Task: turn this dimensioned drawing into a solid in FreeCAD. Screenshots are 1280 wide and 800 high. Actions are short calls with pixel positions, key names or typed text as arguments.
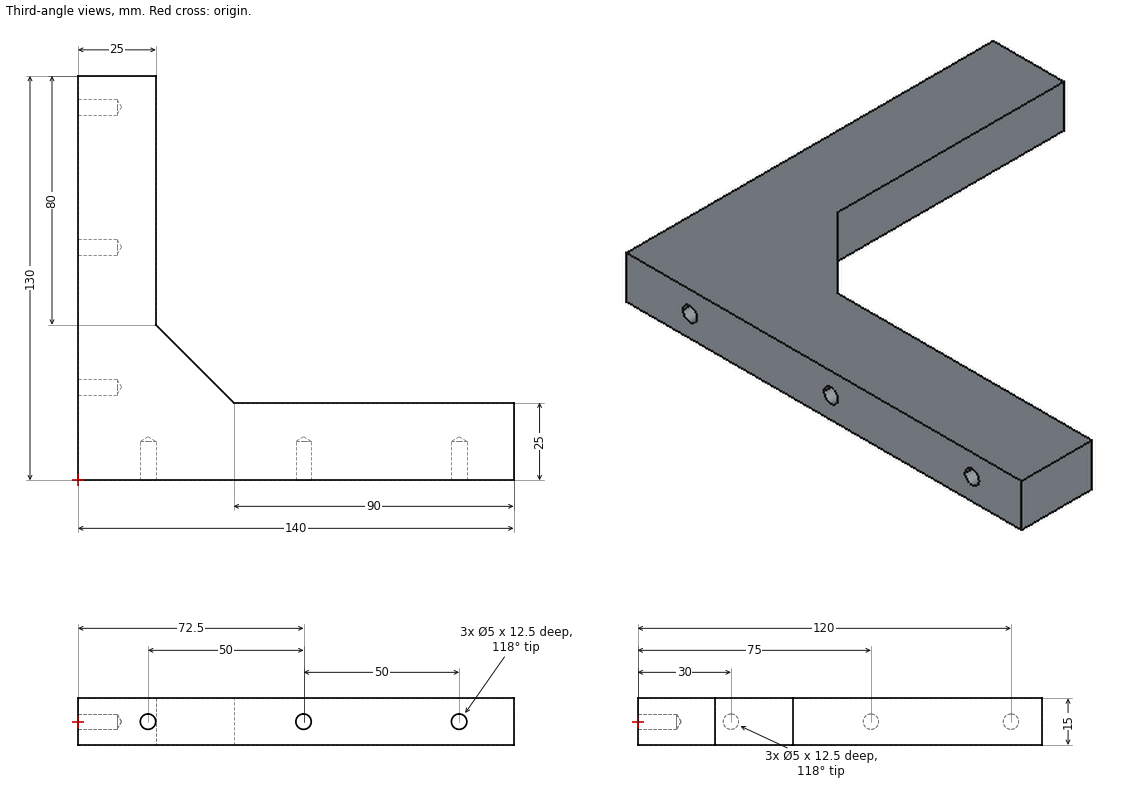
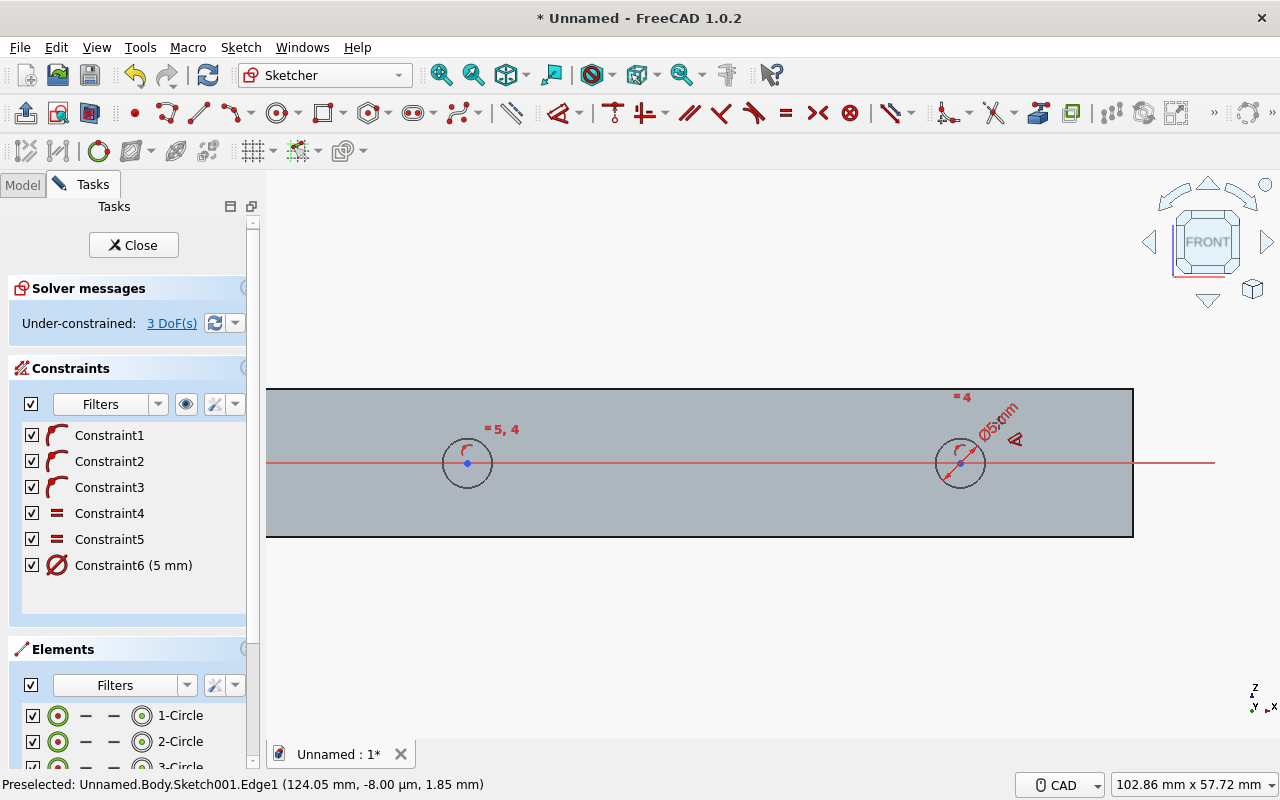
click(960, 463)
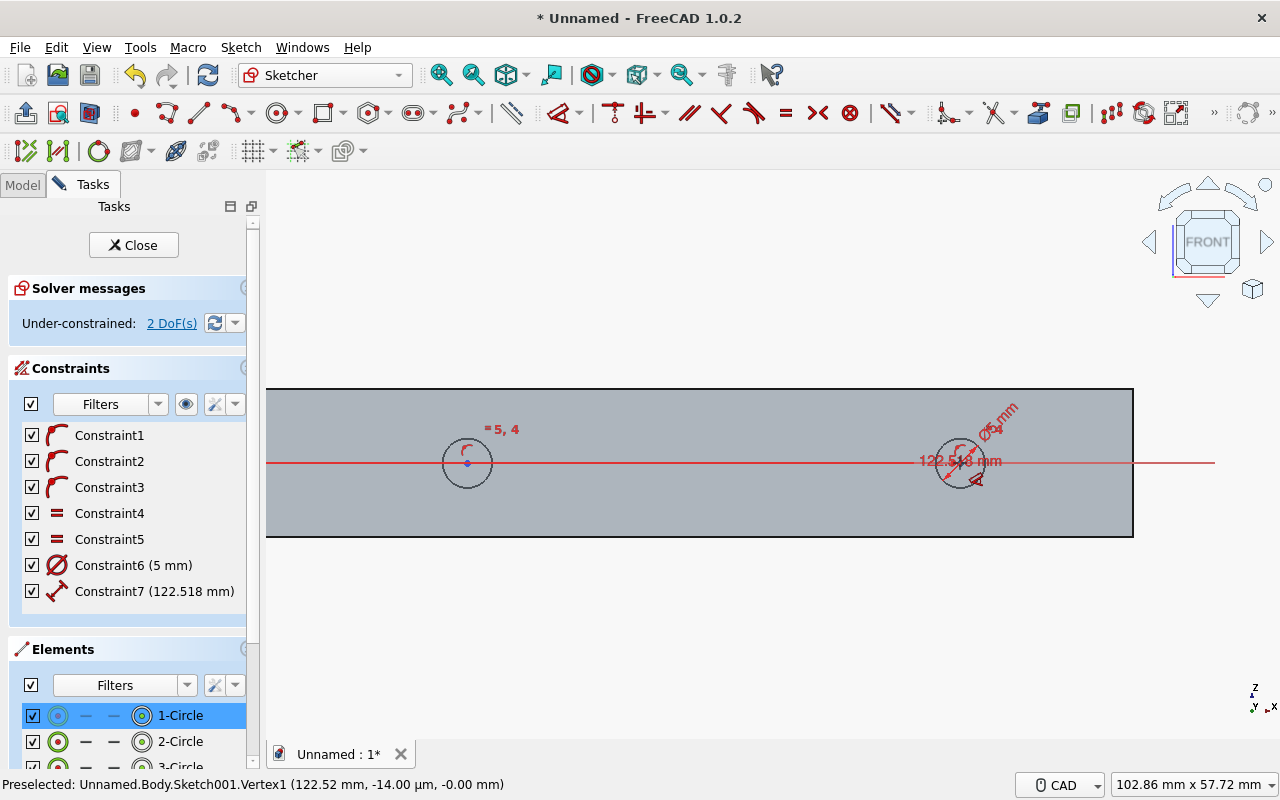
click(467, 463)
click(714, 497)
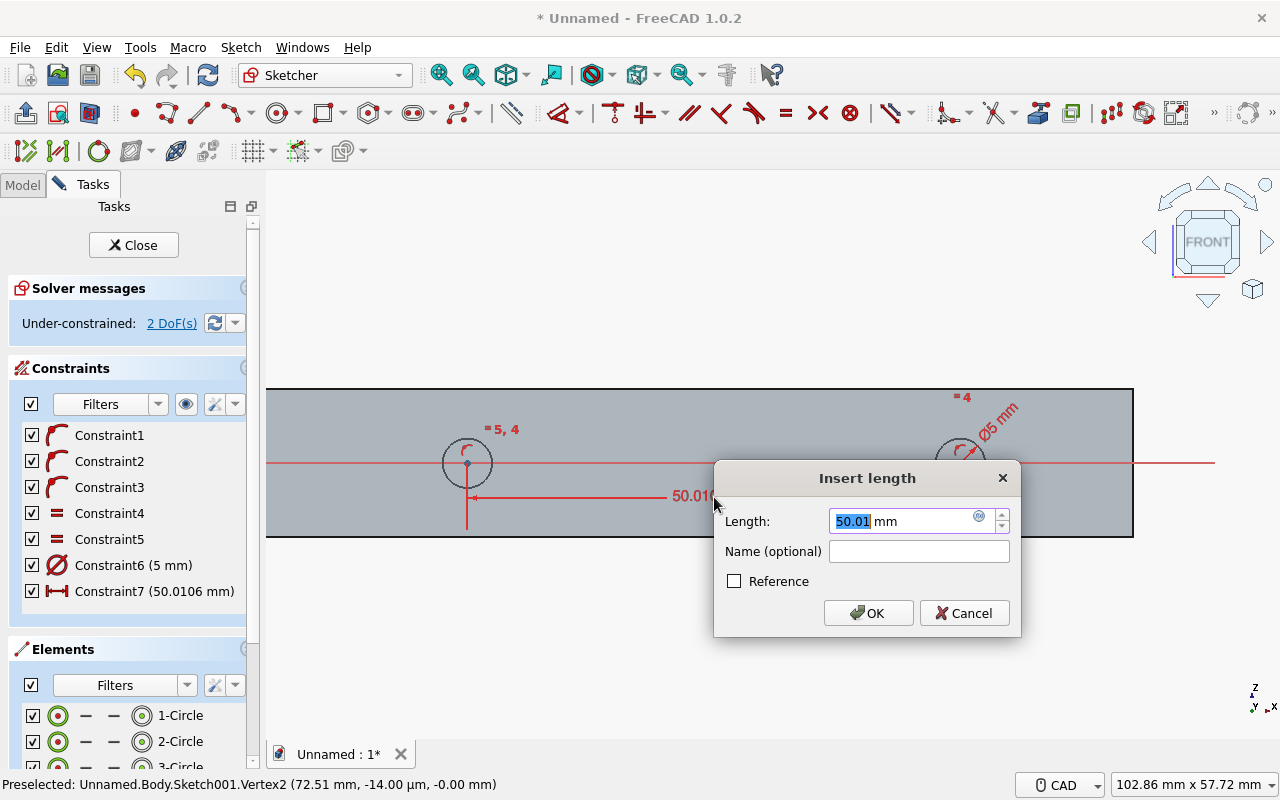
text(50)
key(Return)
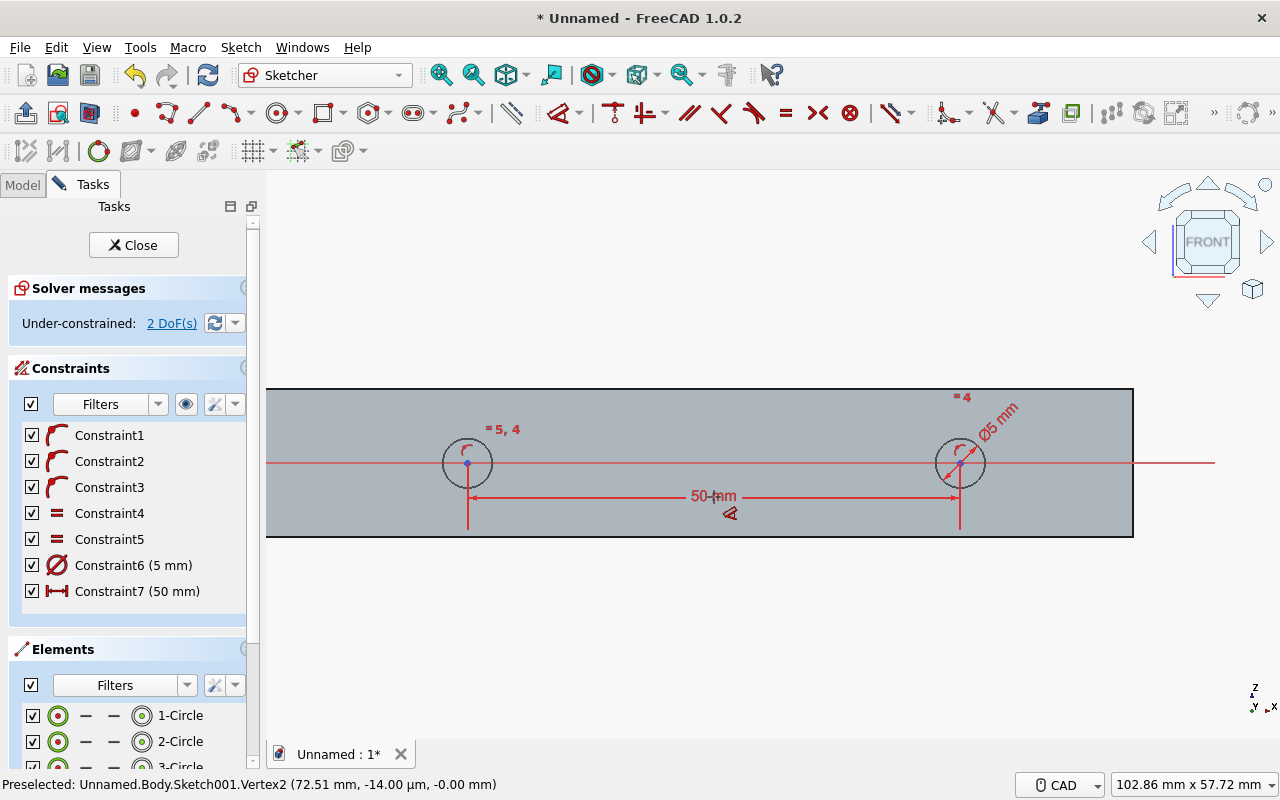
click(468, 463)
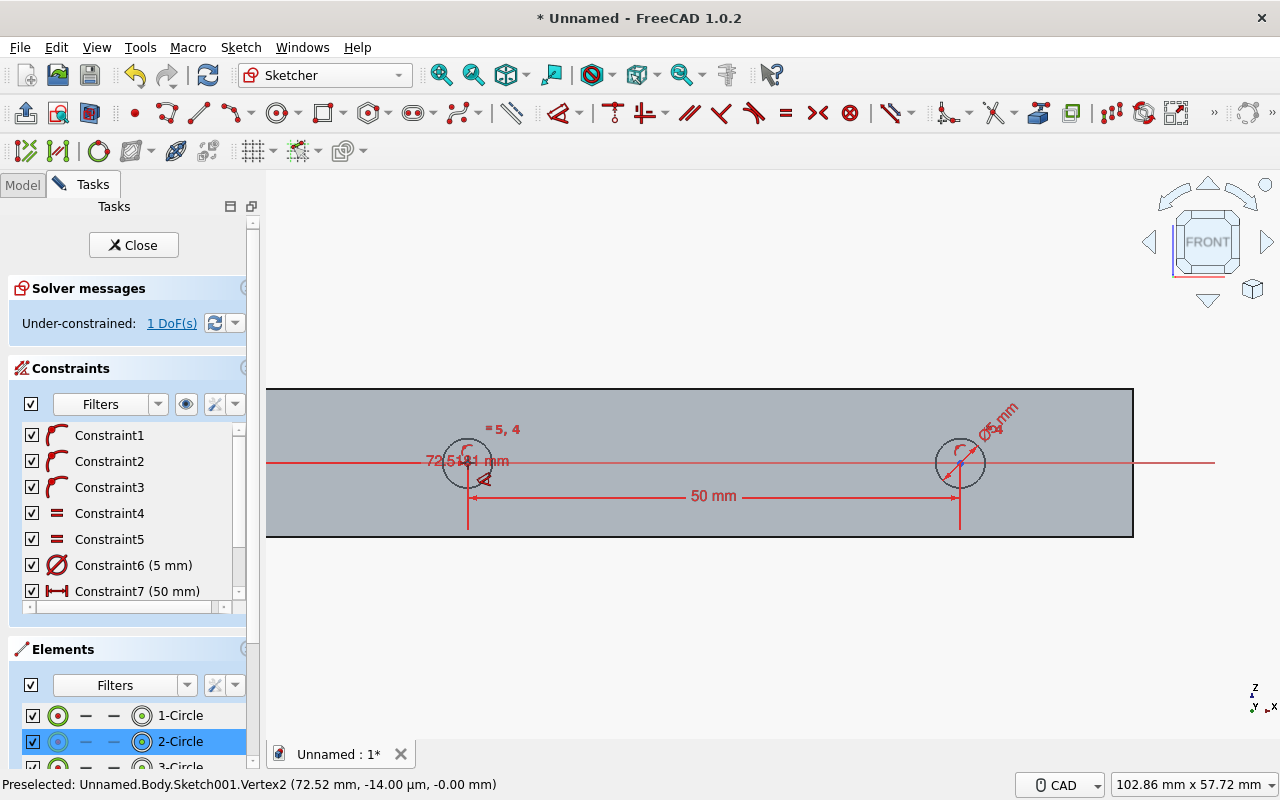
scroll(978, 447, down, 4)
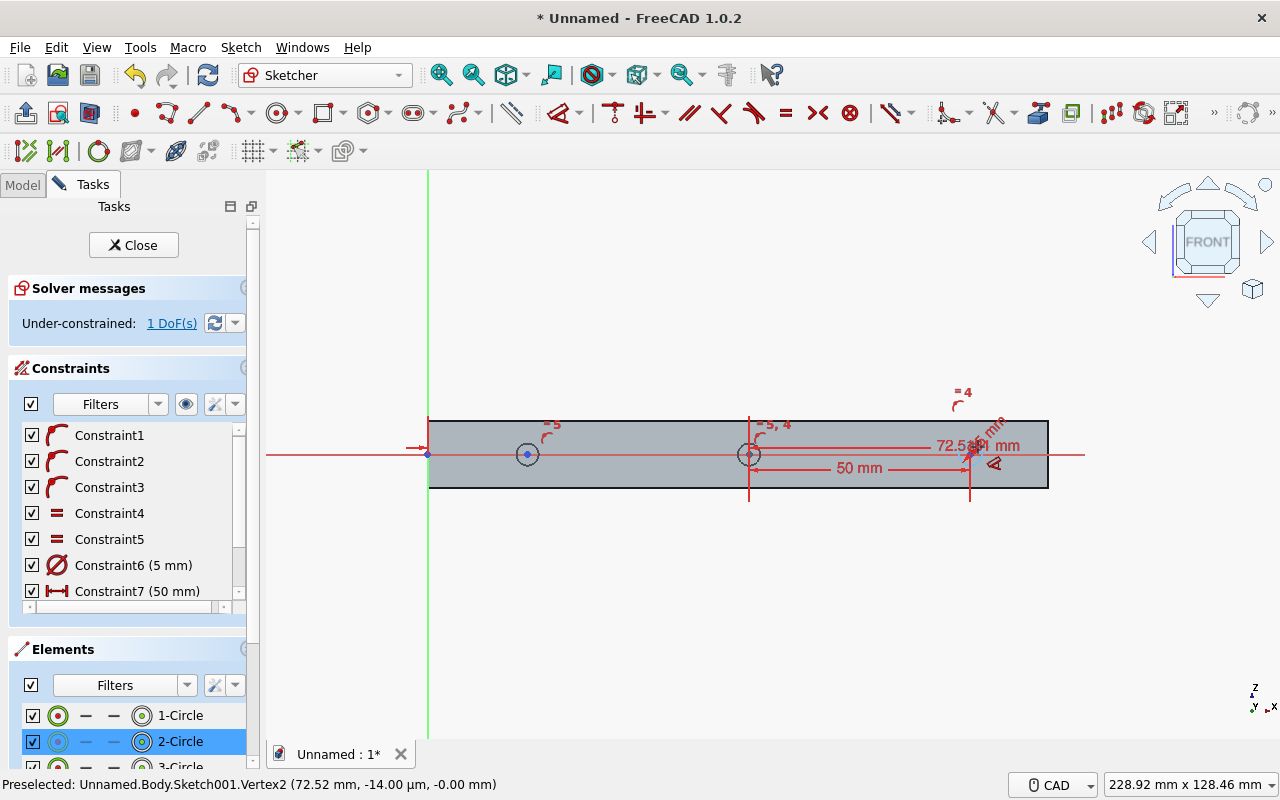
click(528, 455)
click(638, 489)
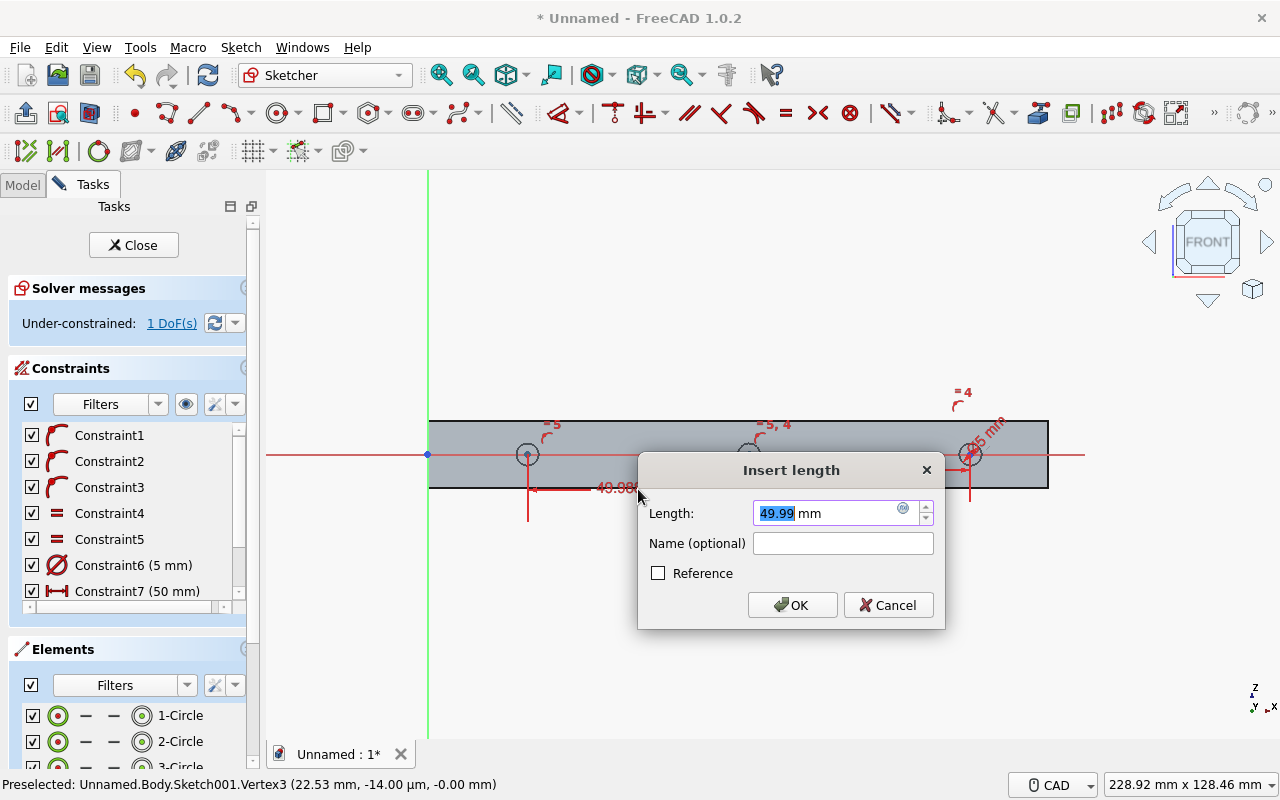
text(50)
key(Return)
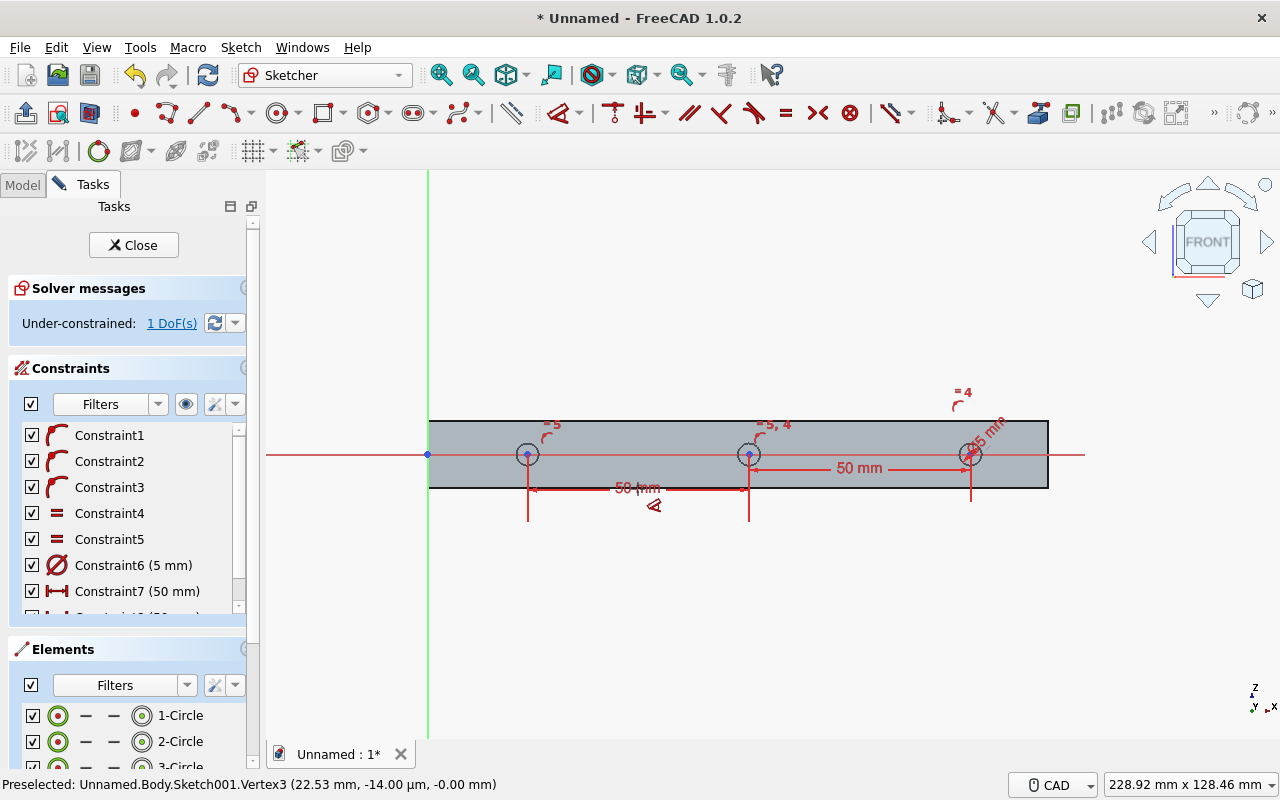
click(749, 455)
click(515, 489)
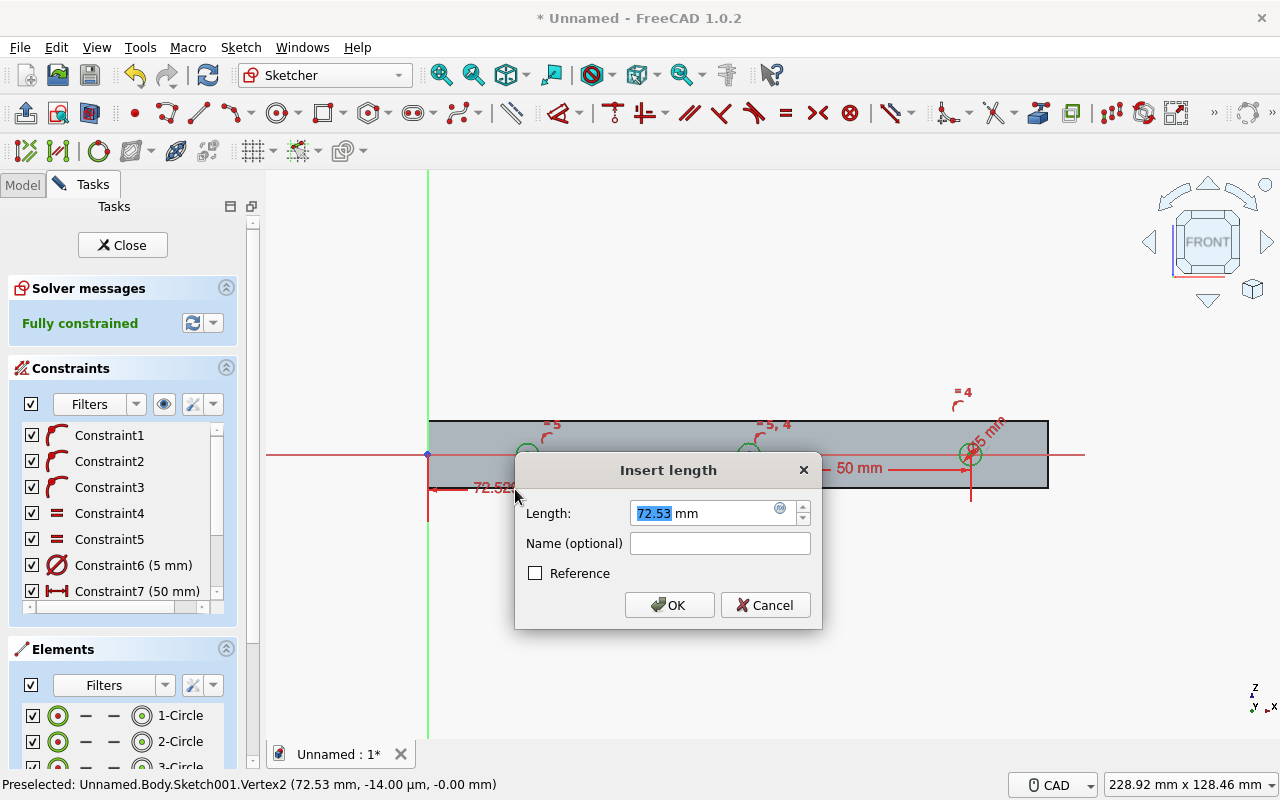
text(72.5)
key(Return)
key(Escape)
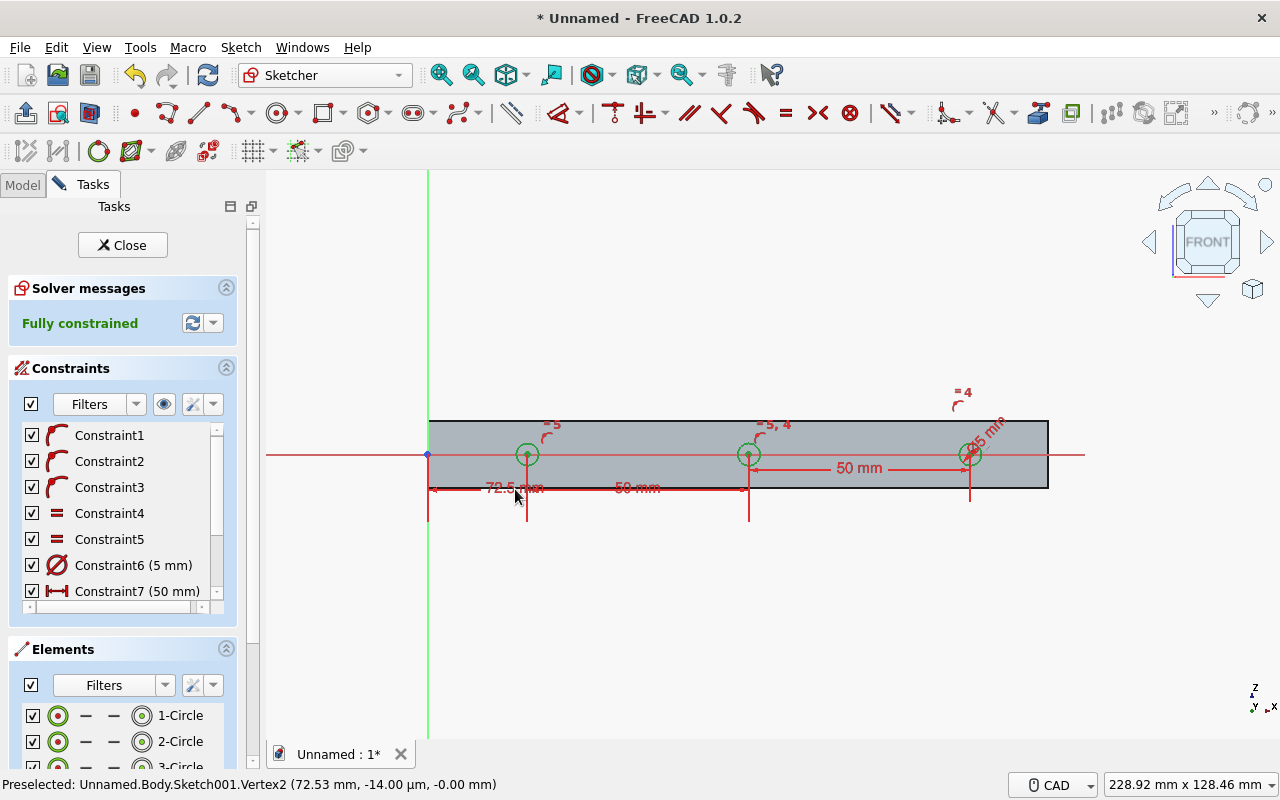
click(123, 245)